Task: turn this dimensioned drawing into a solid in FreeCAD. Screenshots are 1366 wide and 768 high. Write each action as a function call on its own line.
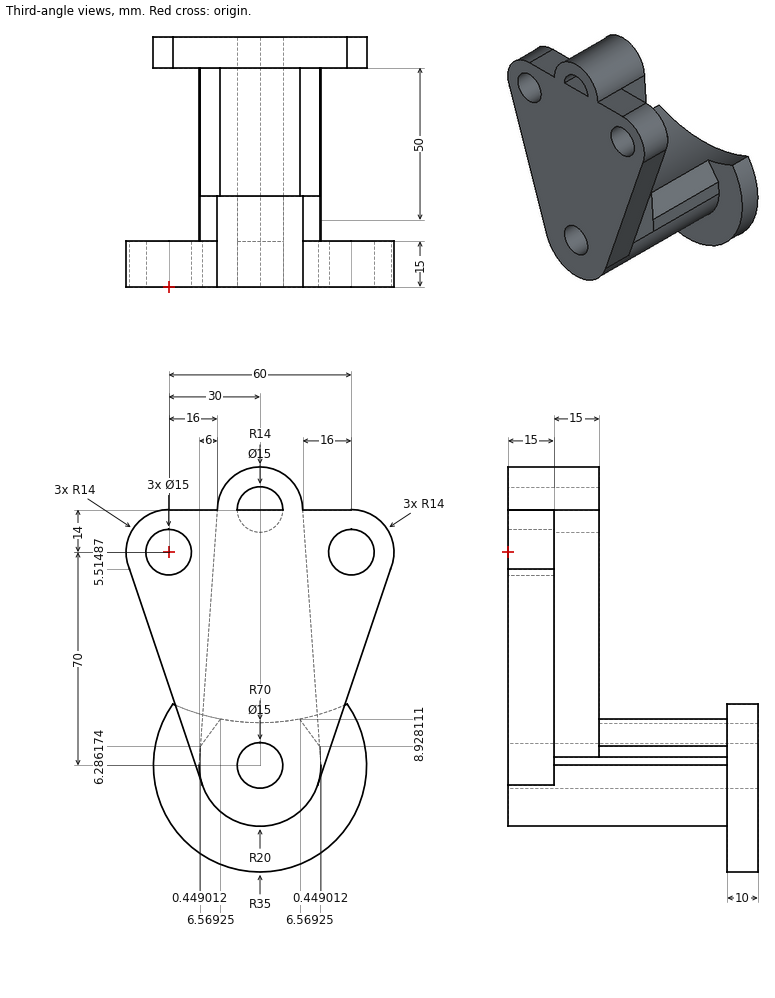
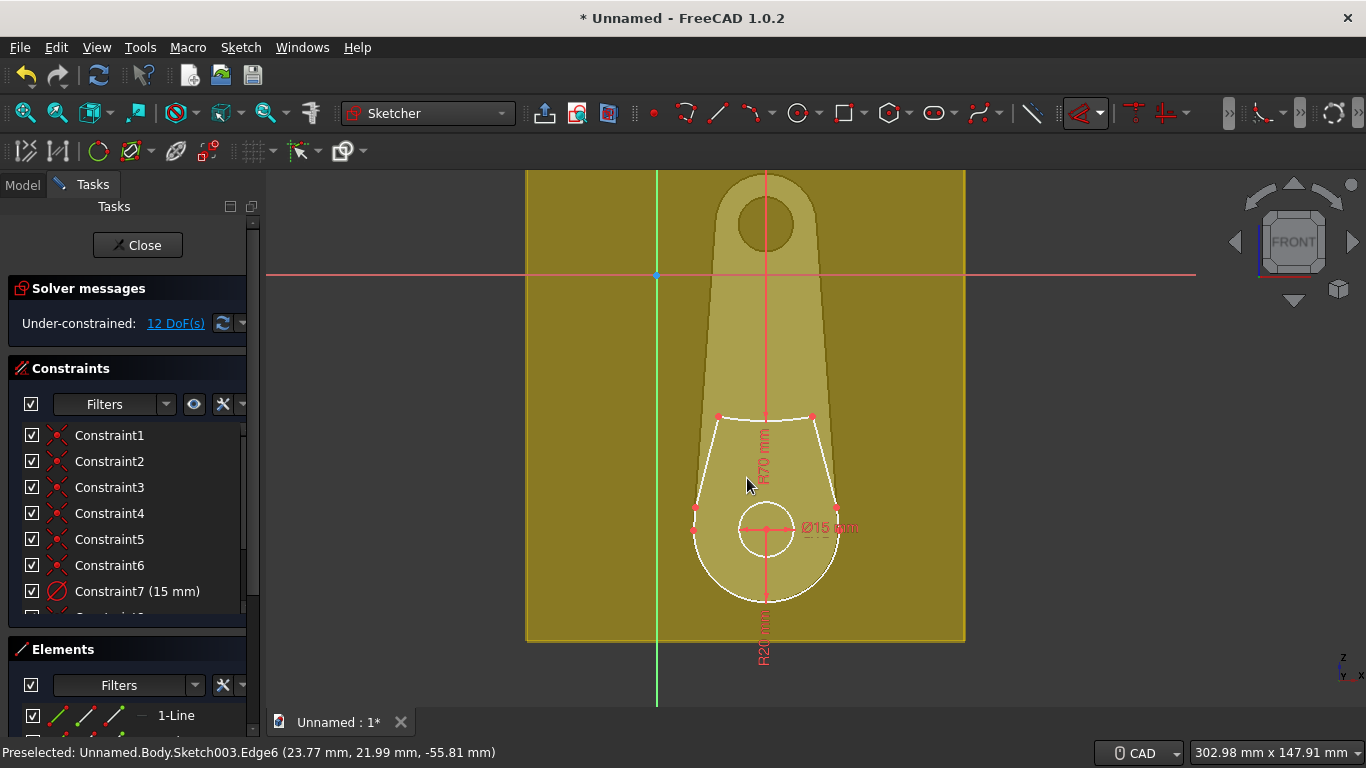
click(766, 530)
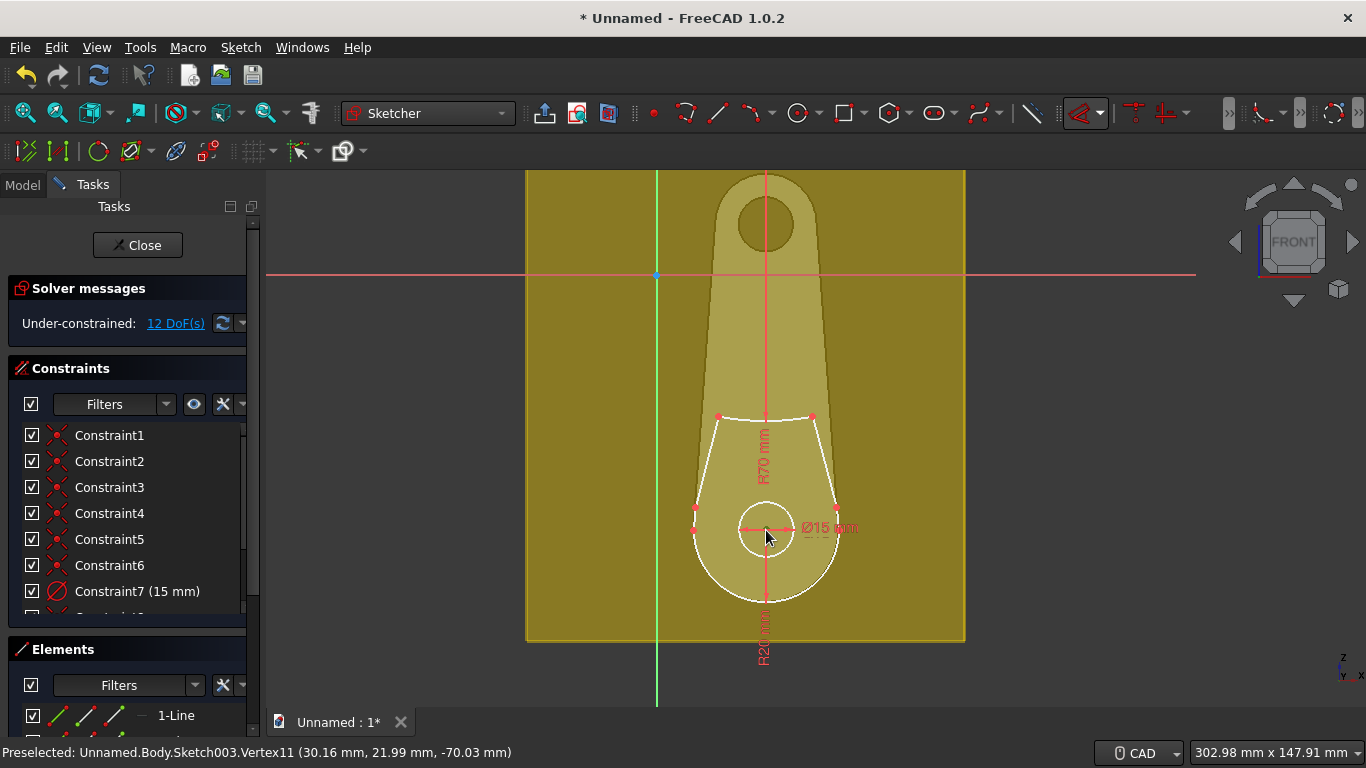
key(l)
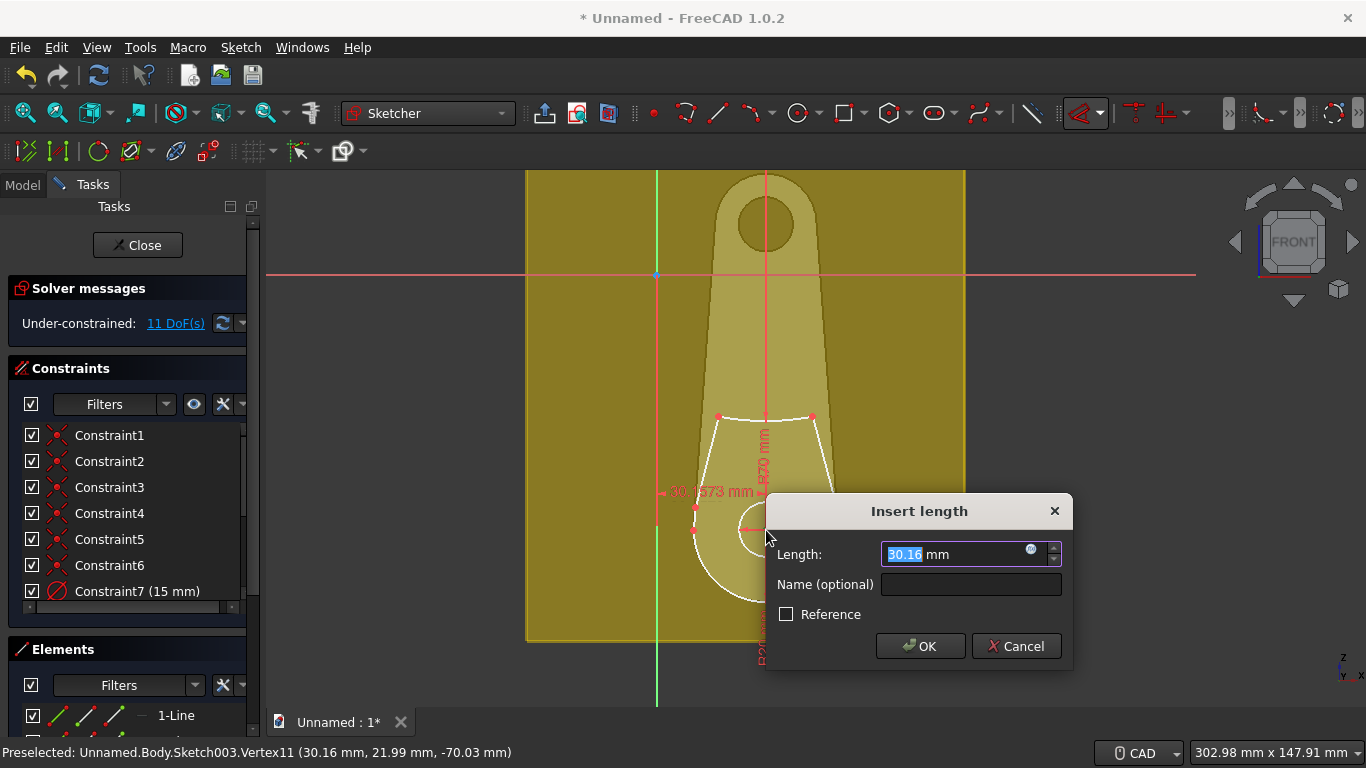
text(30)
key(Return)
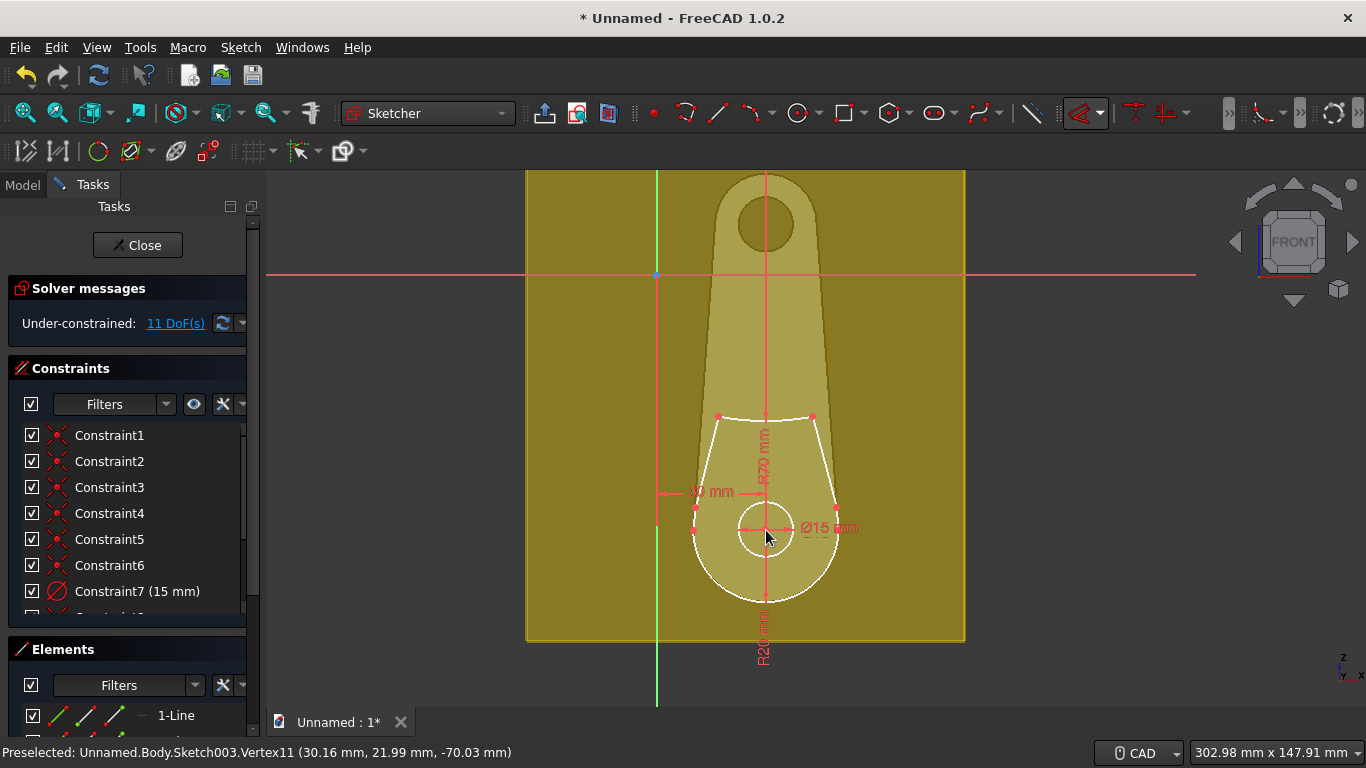
click(766, 530)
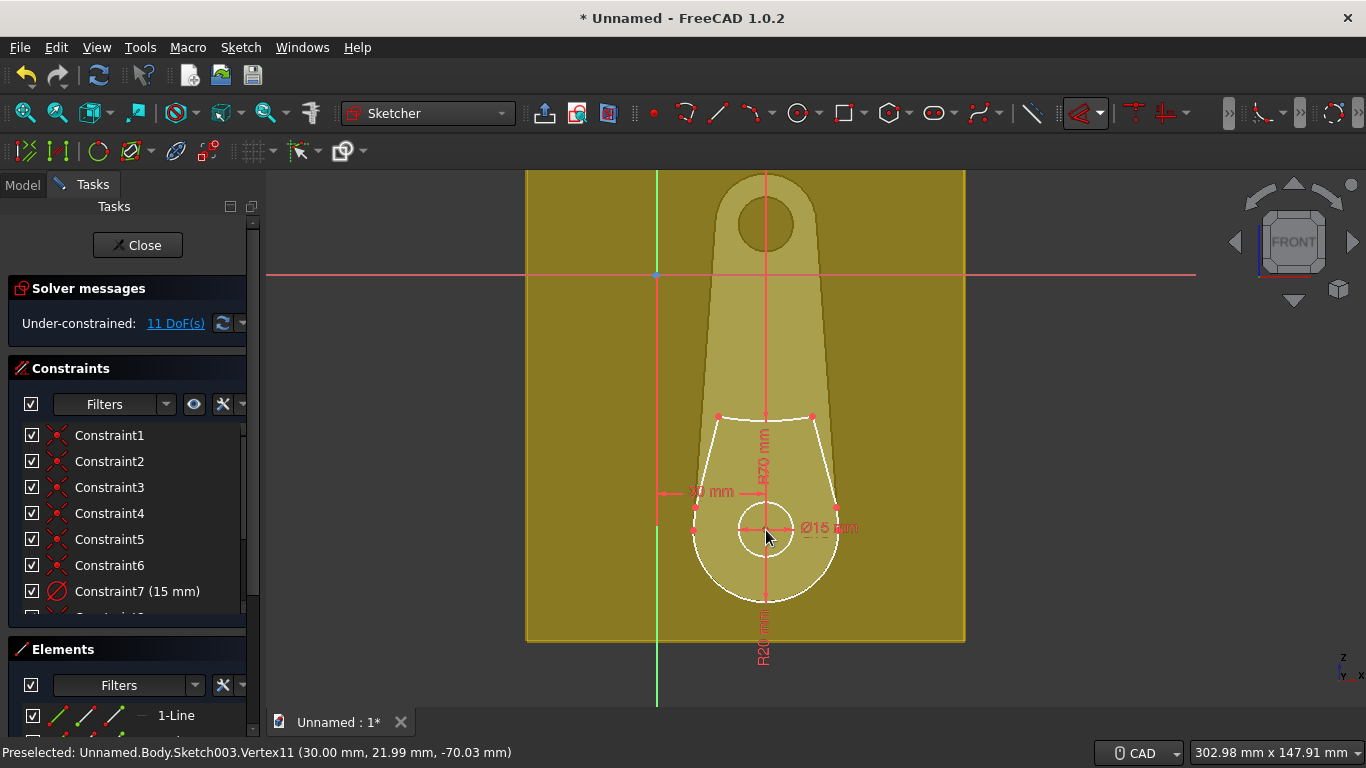
click(1102, 114)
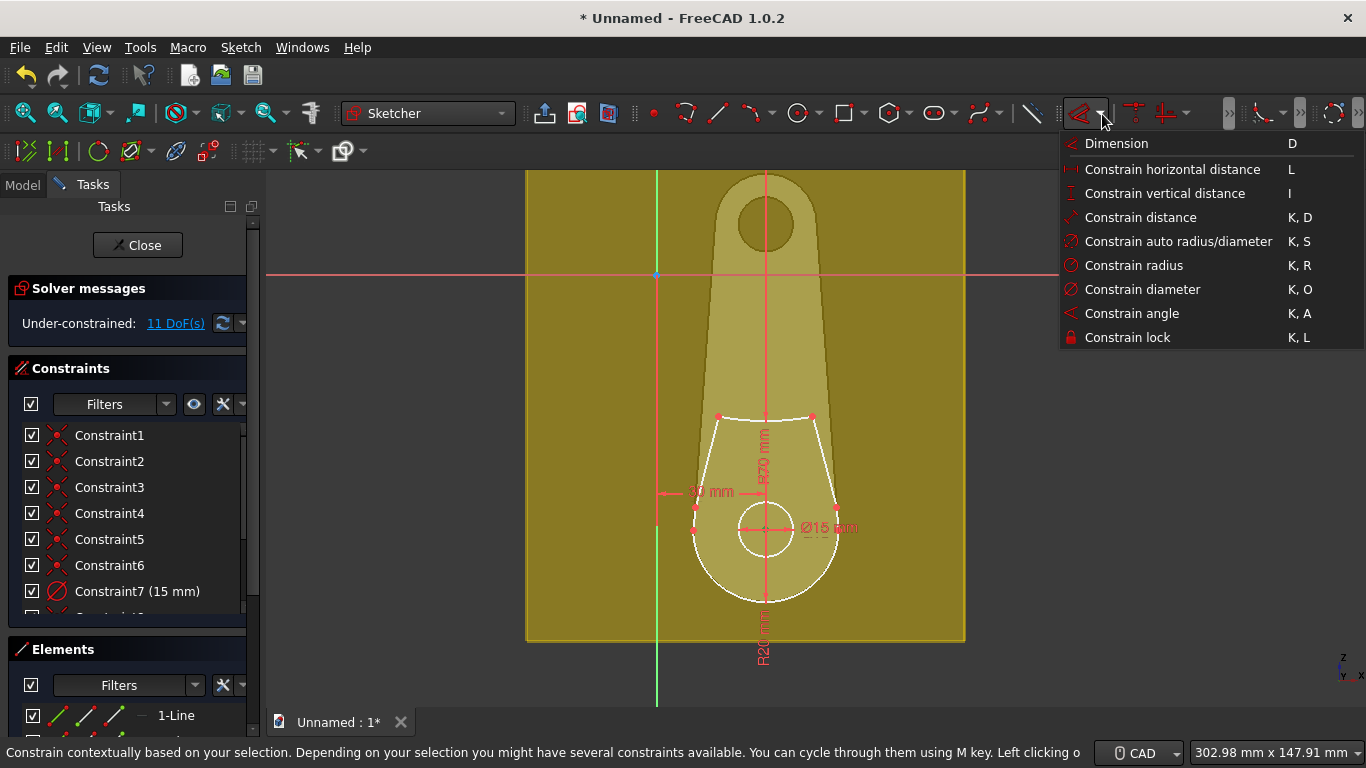
click(1212, 193)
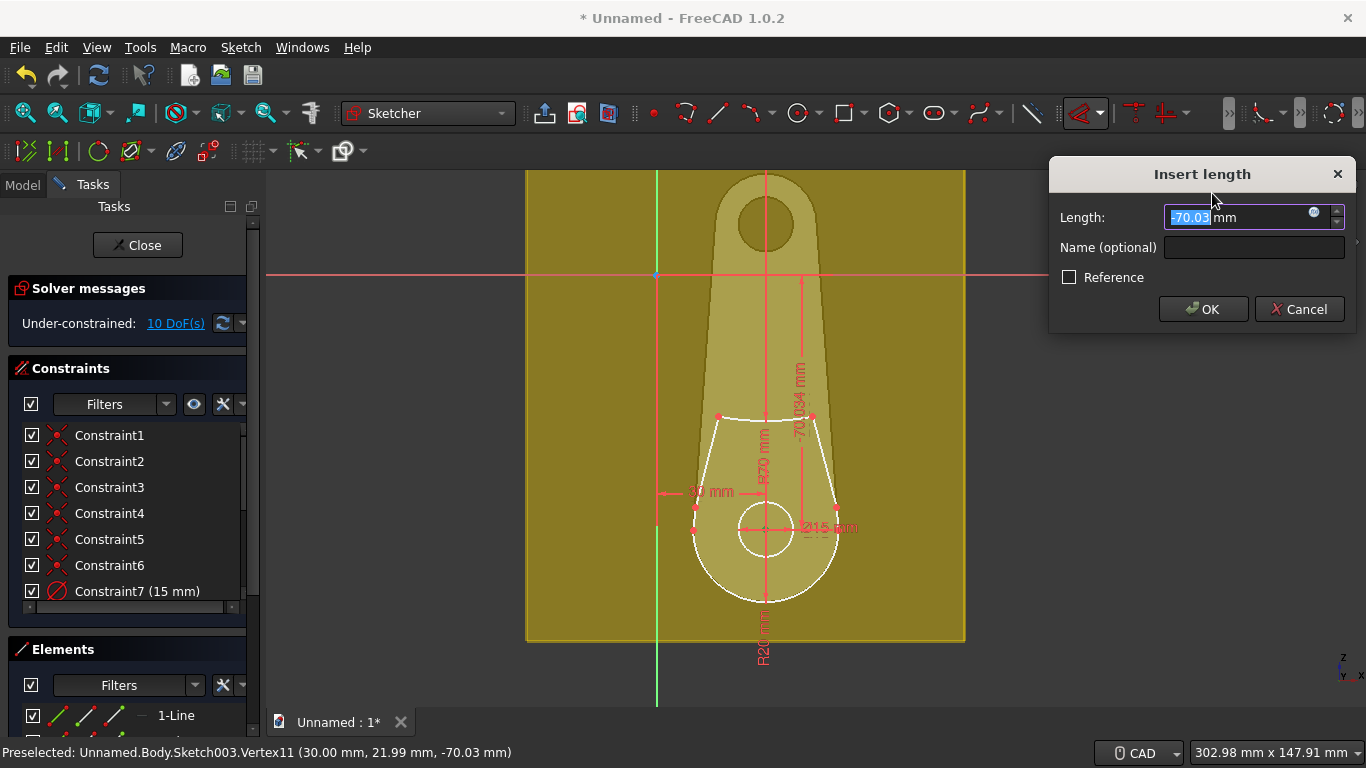
text(-70)
key(Return)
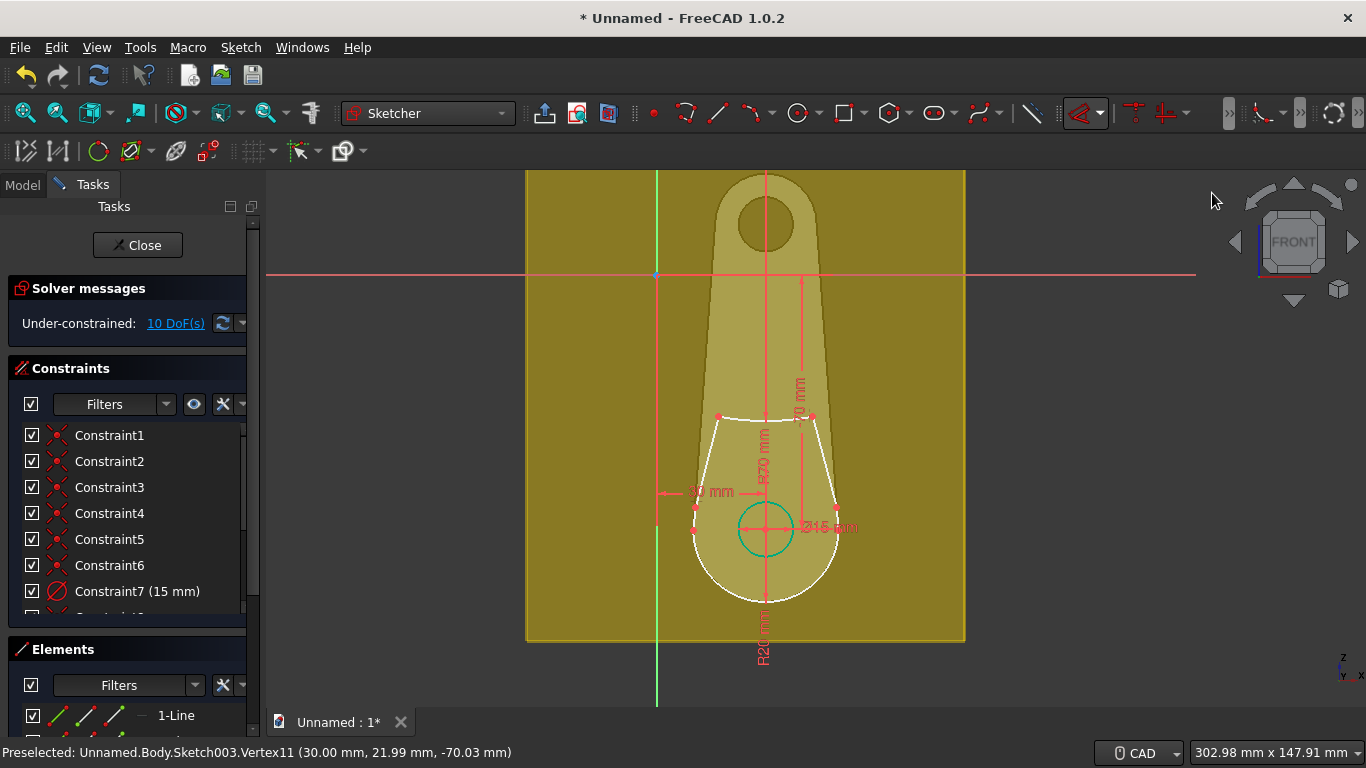
click(838, 530)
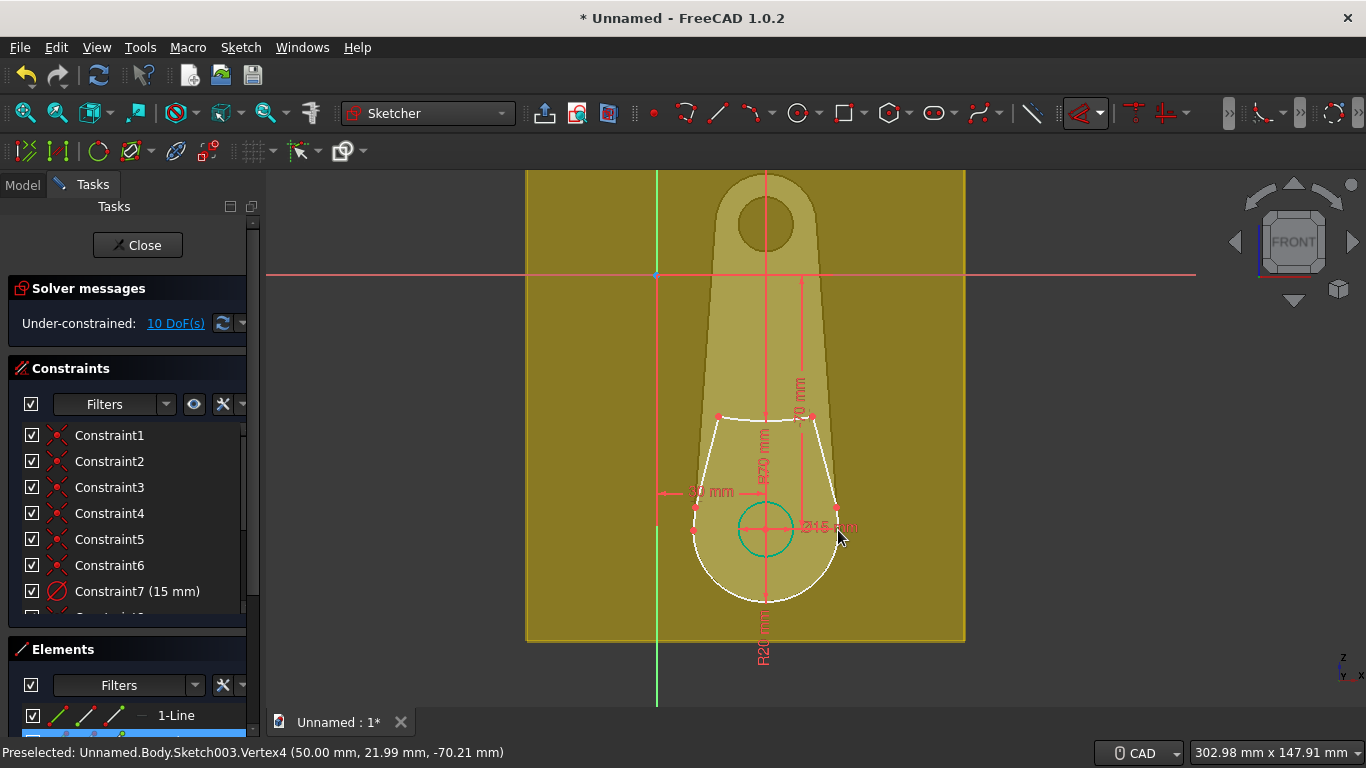
click(1102, 114)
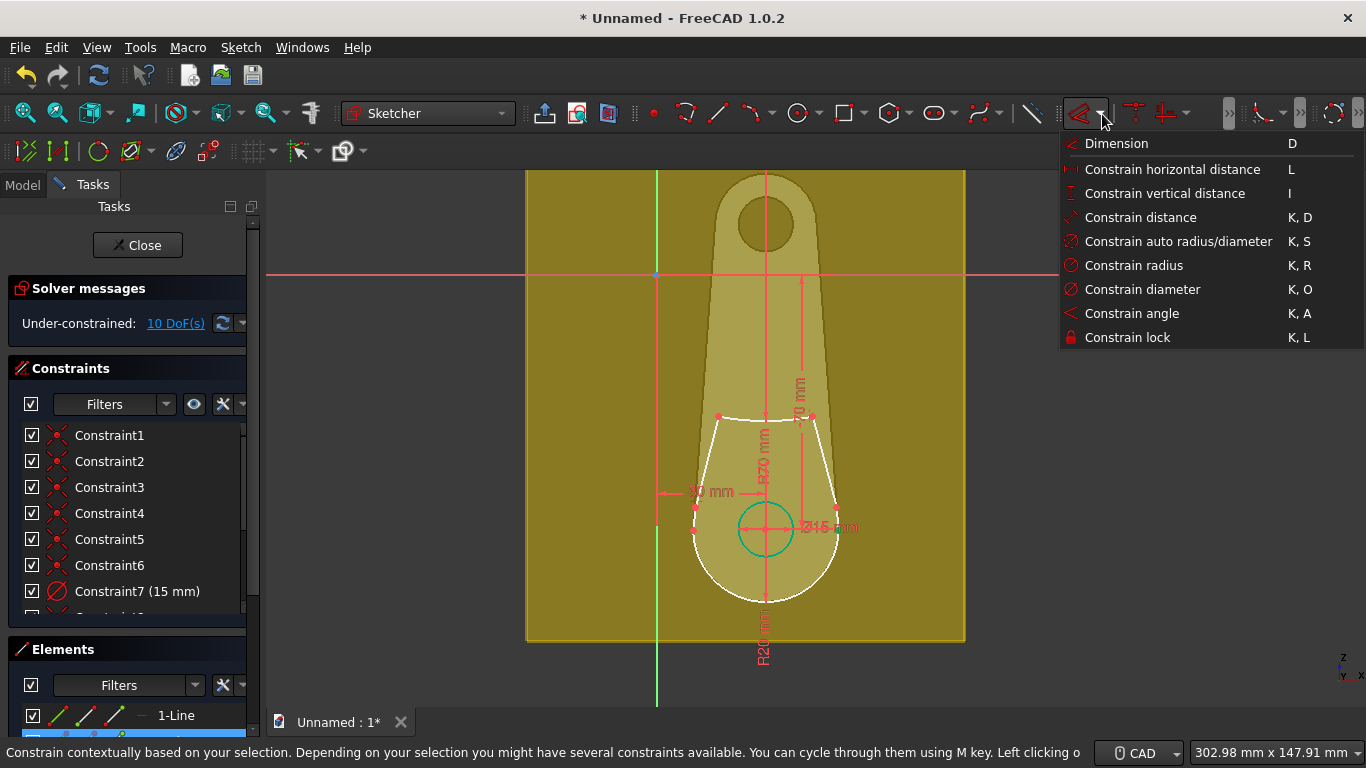
click(1212, 193)